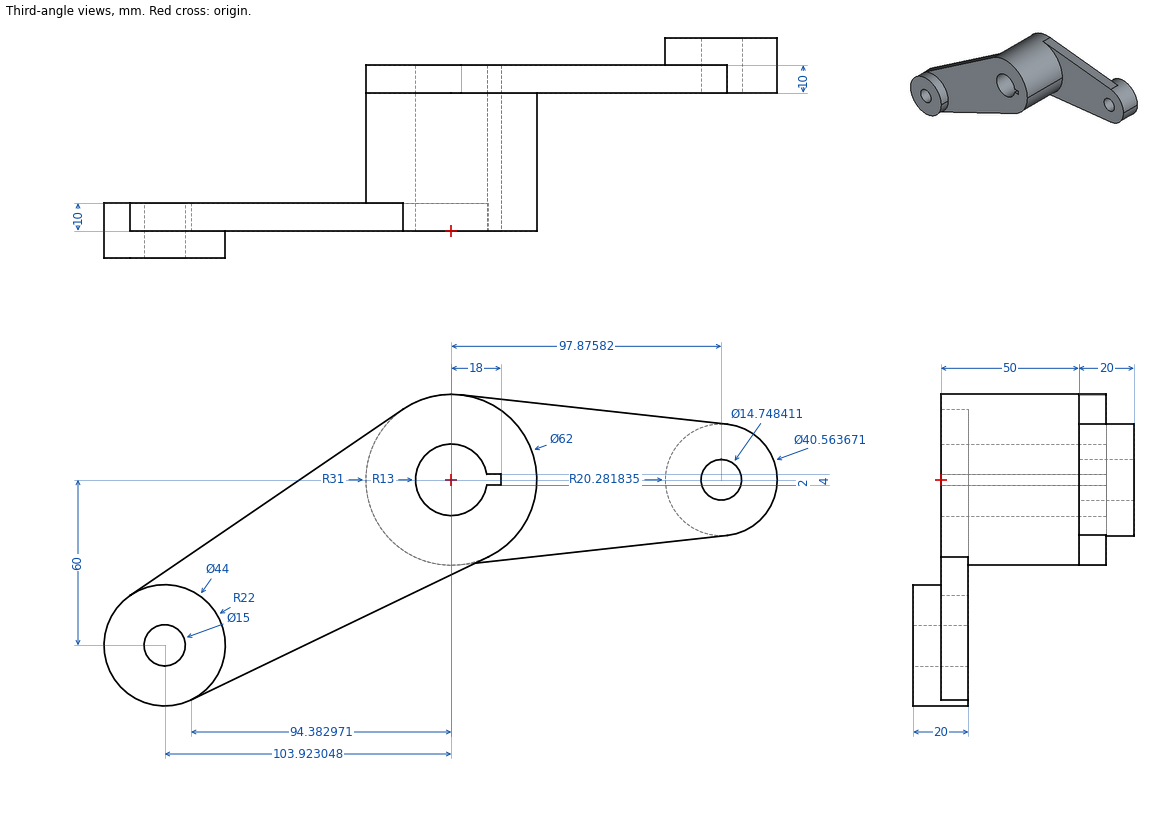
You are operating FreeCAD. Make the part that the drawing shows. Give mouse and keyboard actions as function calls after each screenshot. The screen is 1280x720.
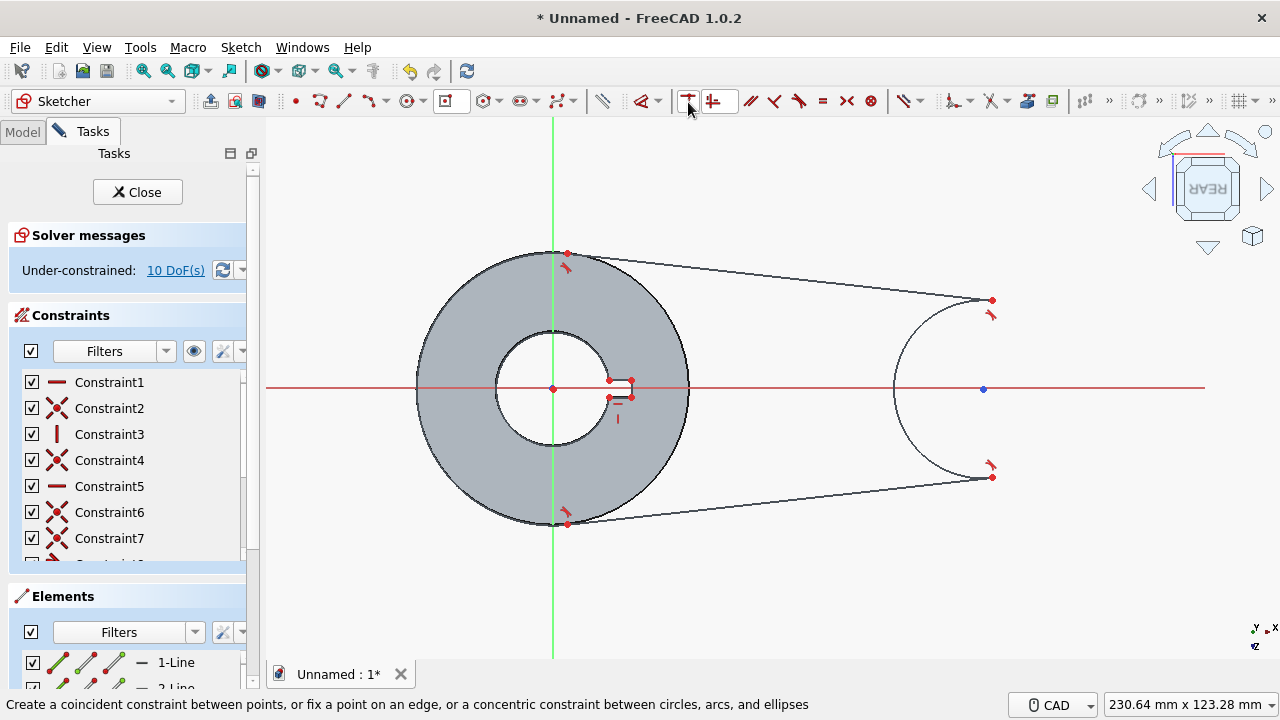
drag(543, 378, 563, 399)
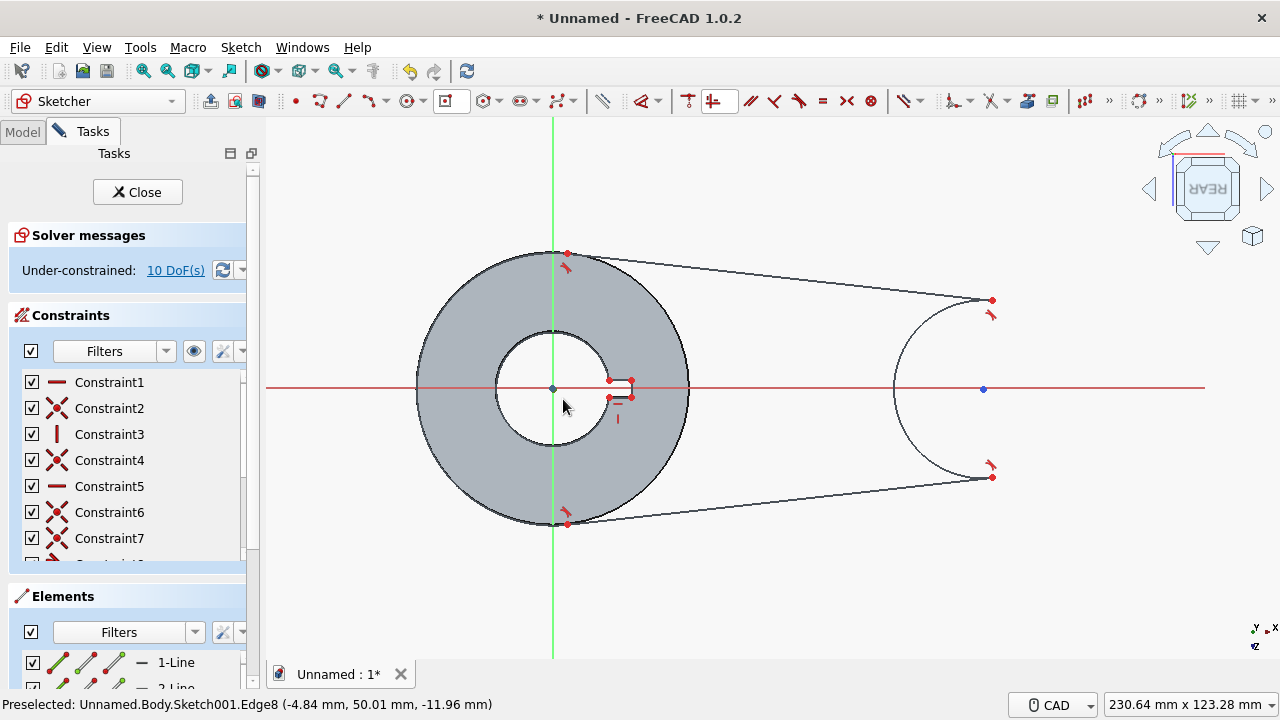
key(c)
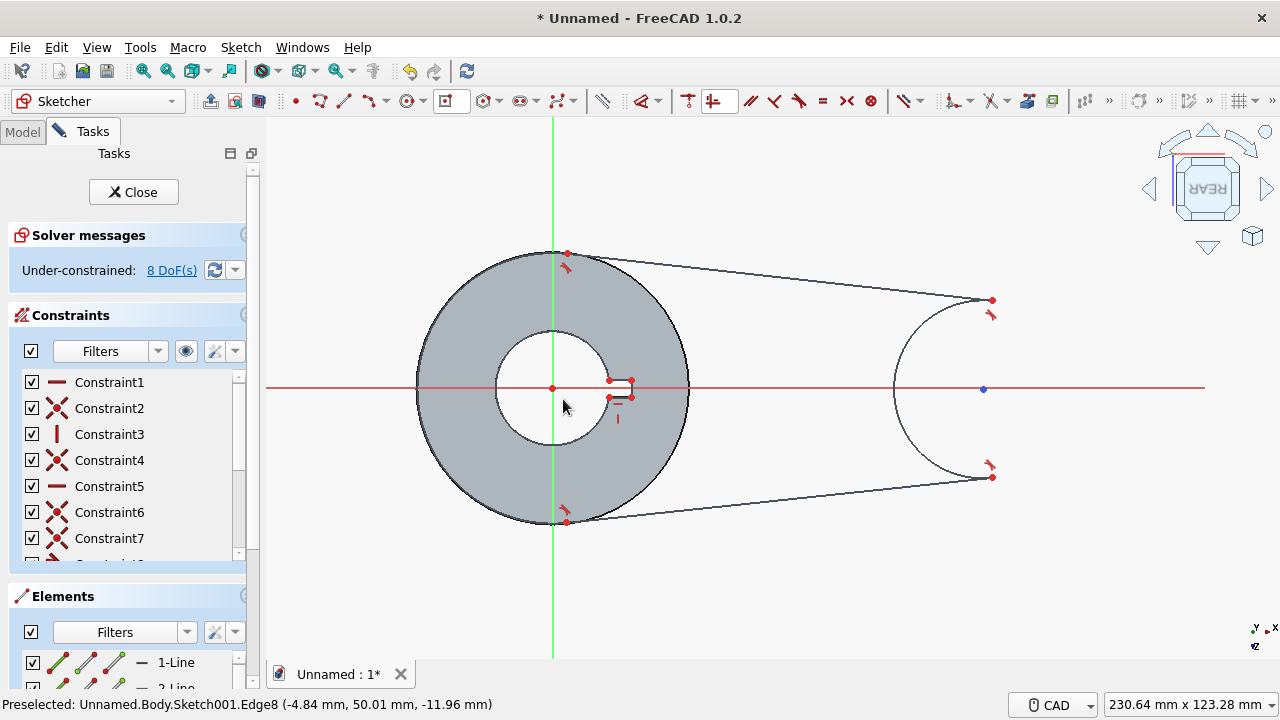
click(983, 389)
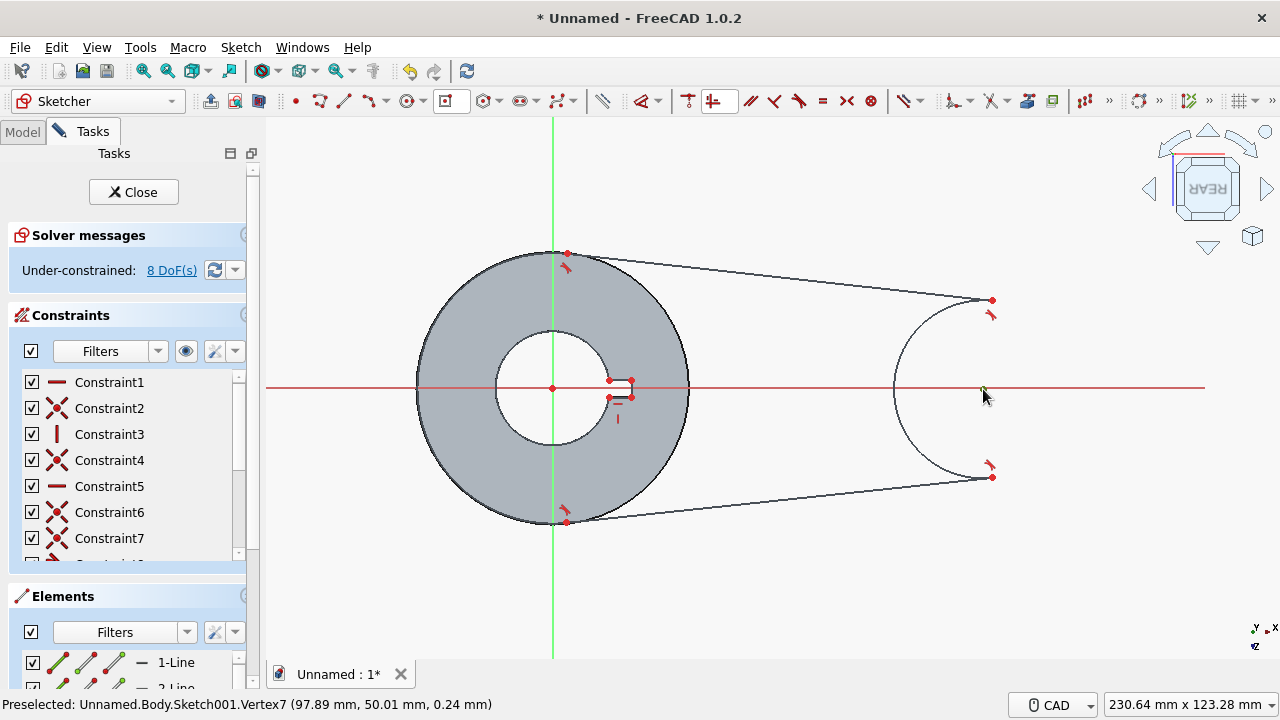
click(353, 388)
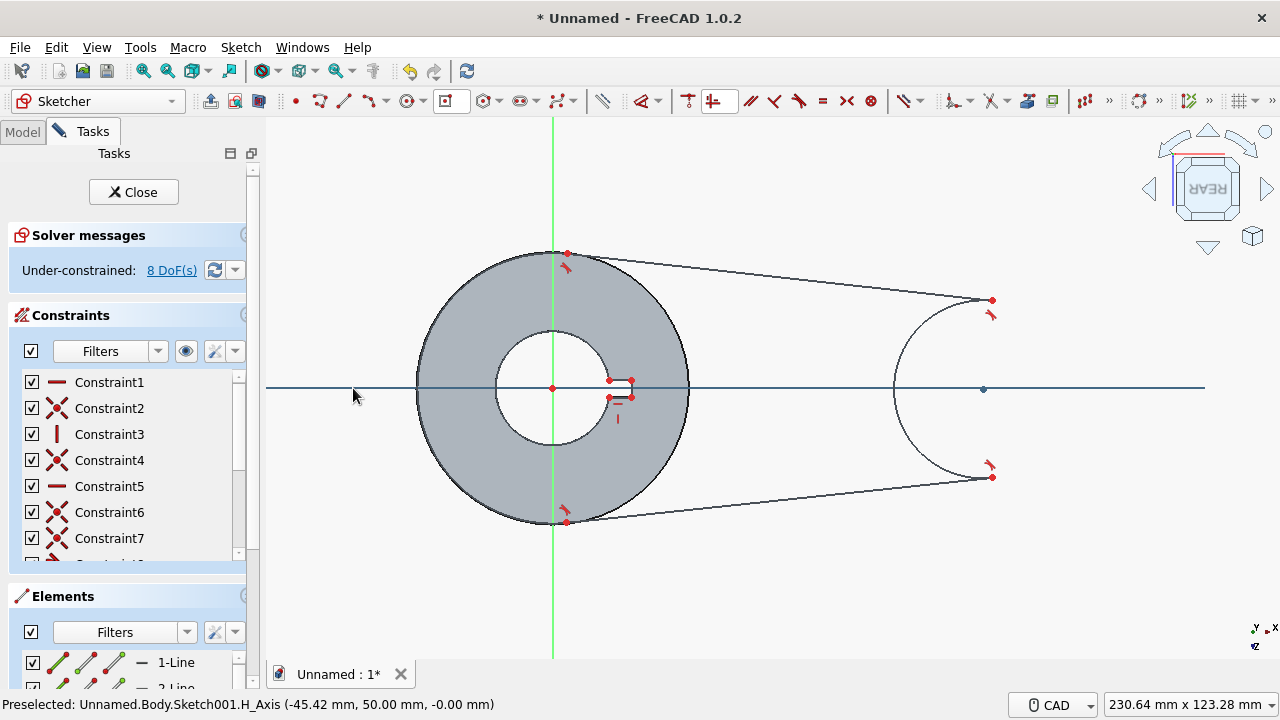
key(c)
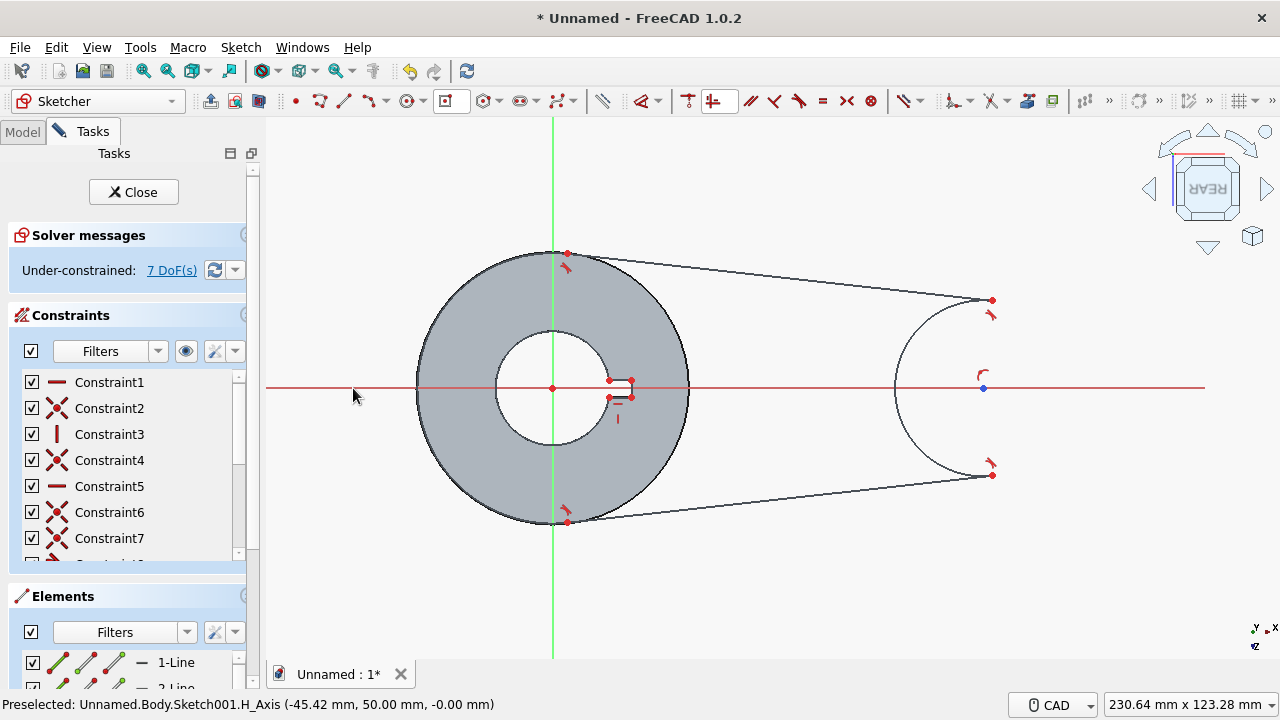
click(642, 102)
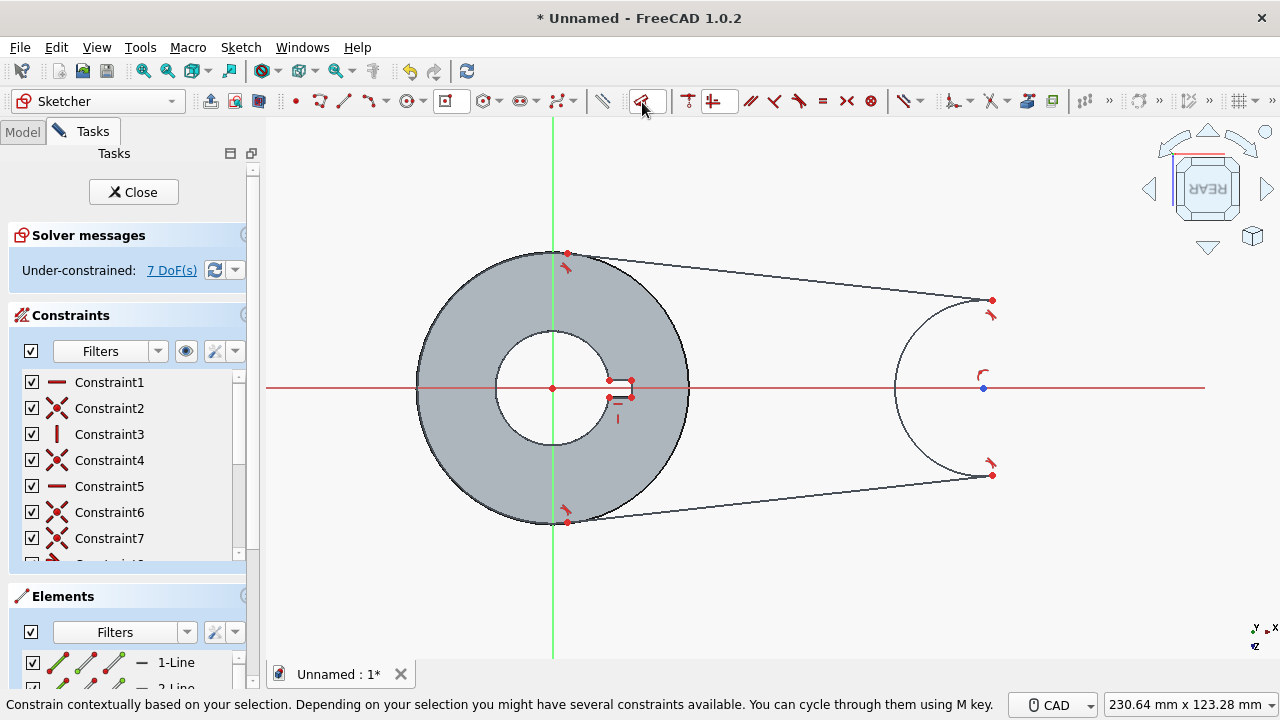
click(914, 334)
click(889, 314)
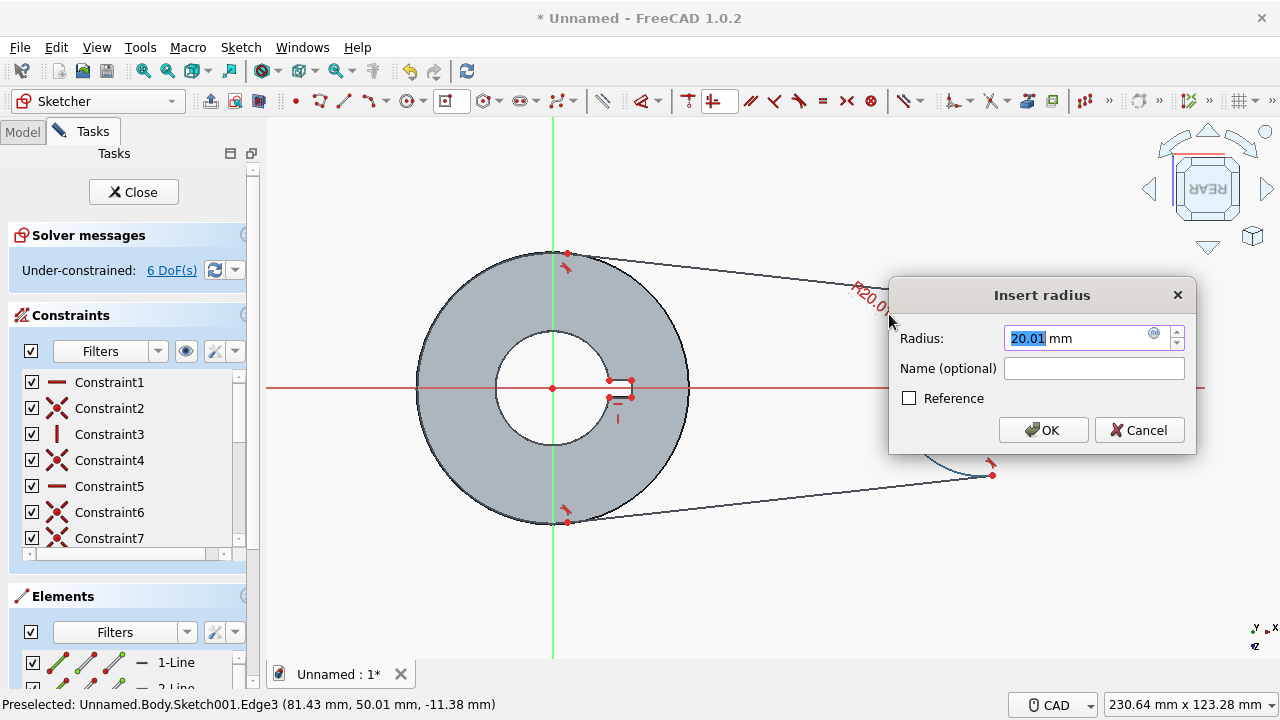
text(20.281835)
key(Return)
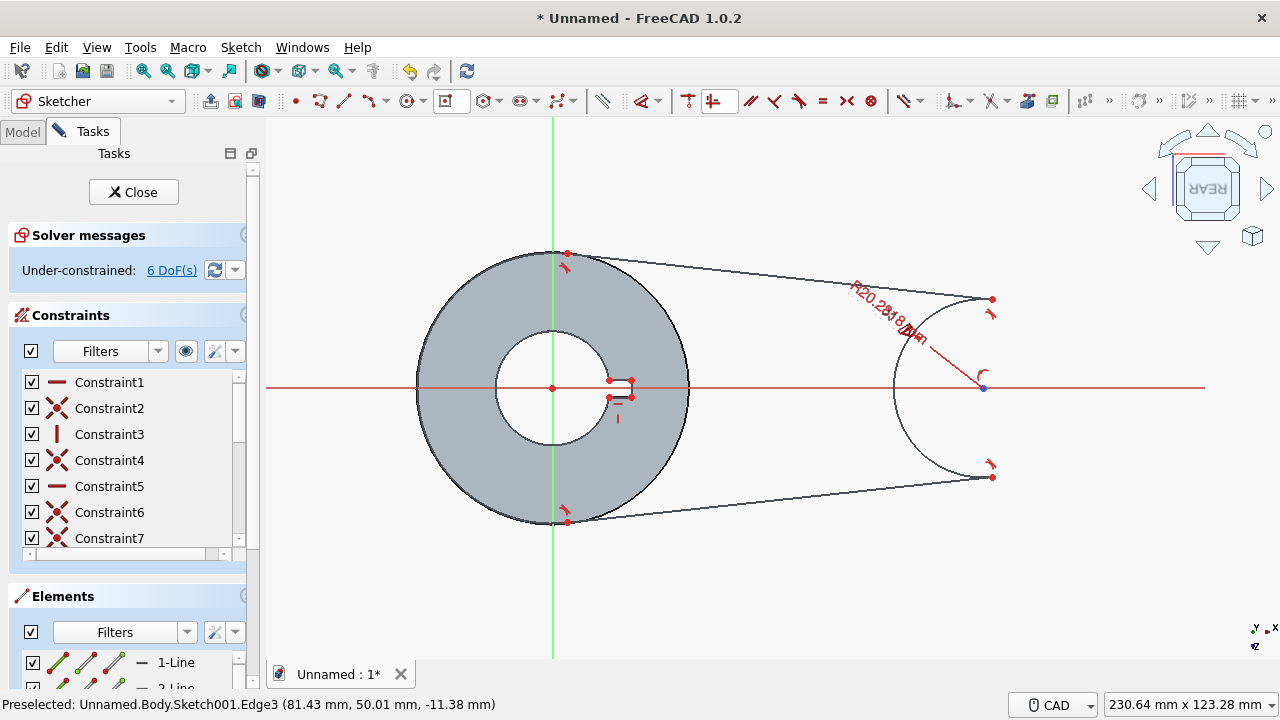
click(447, 304)
click(422, 284)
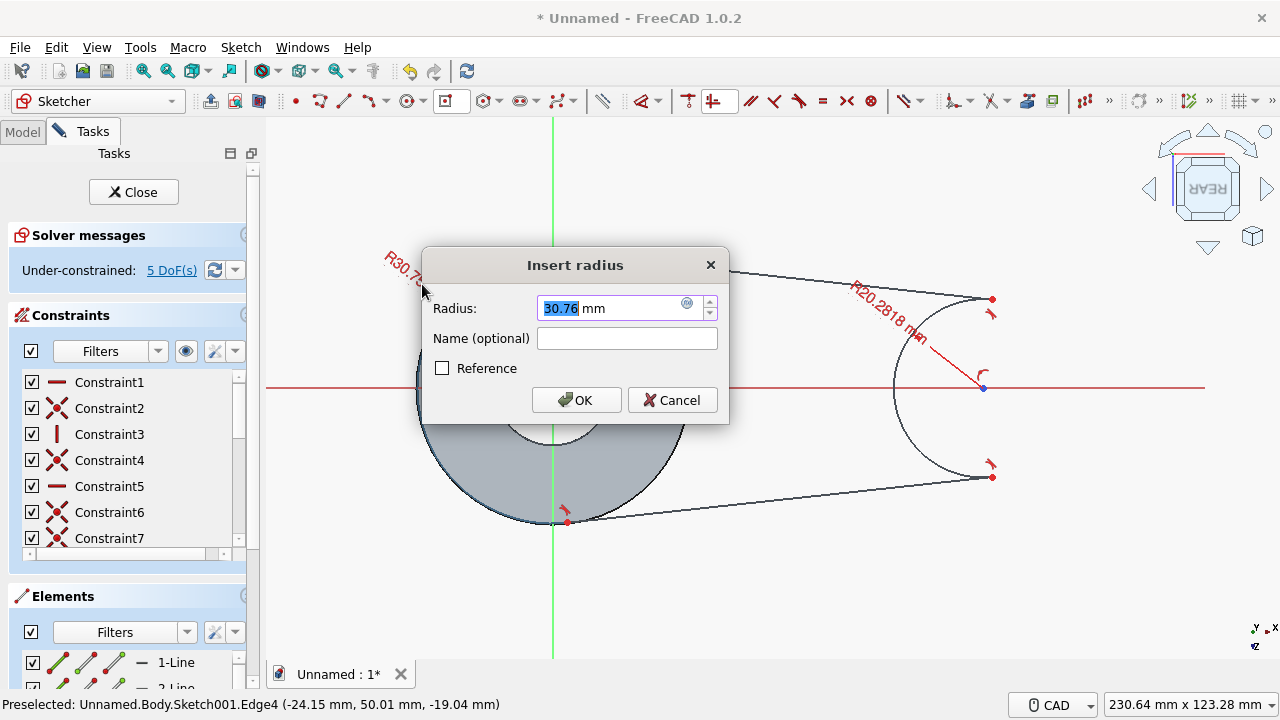
text(31)
key(Return)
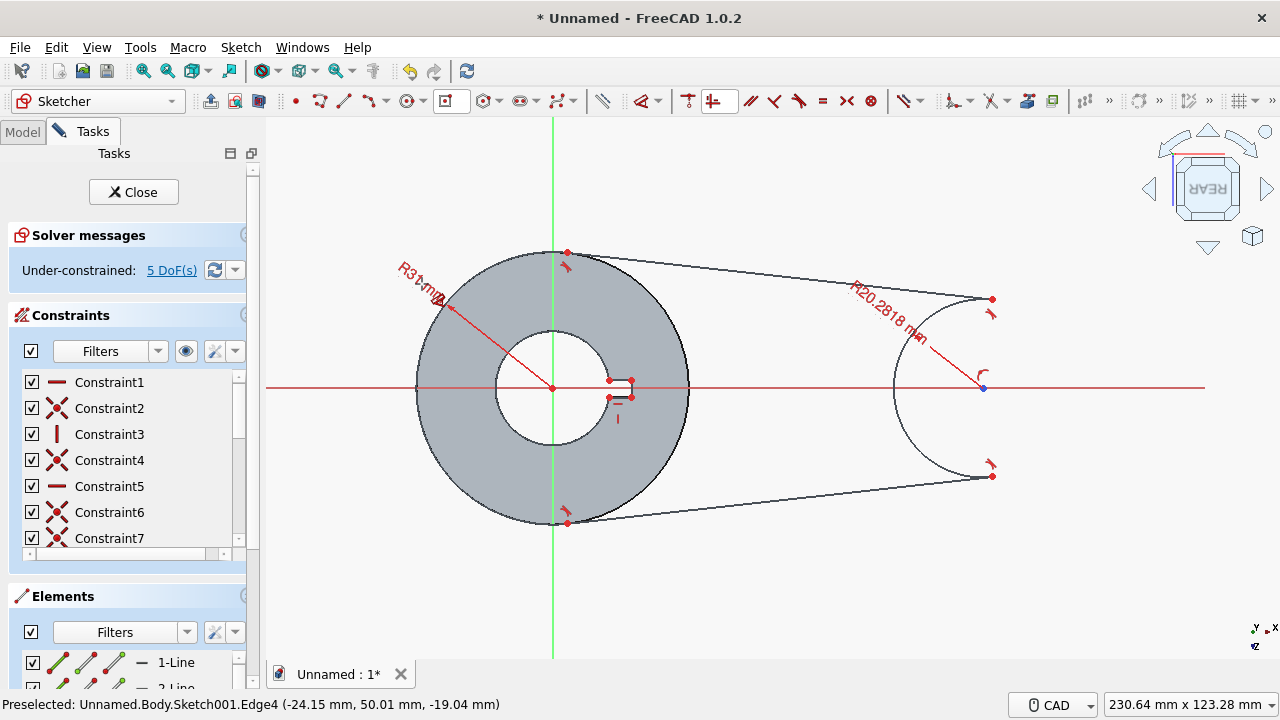
click(532, 335)
click(520, 305)